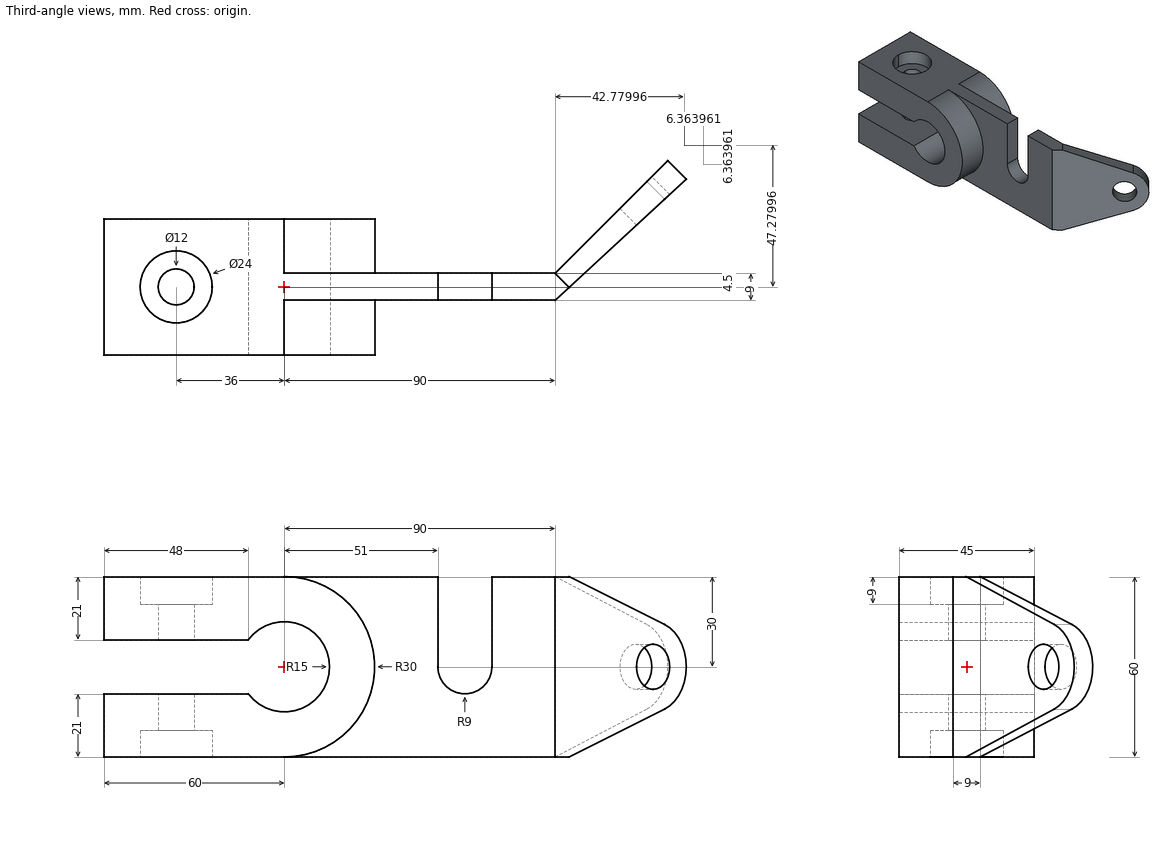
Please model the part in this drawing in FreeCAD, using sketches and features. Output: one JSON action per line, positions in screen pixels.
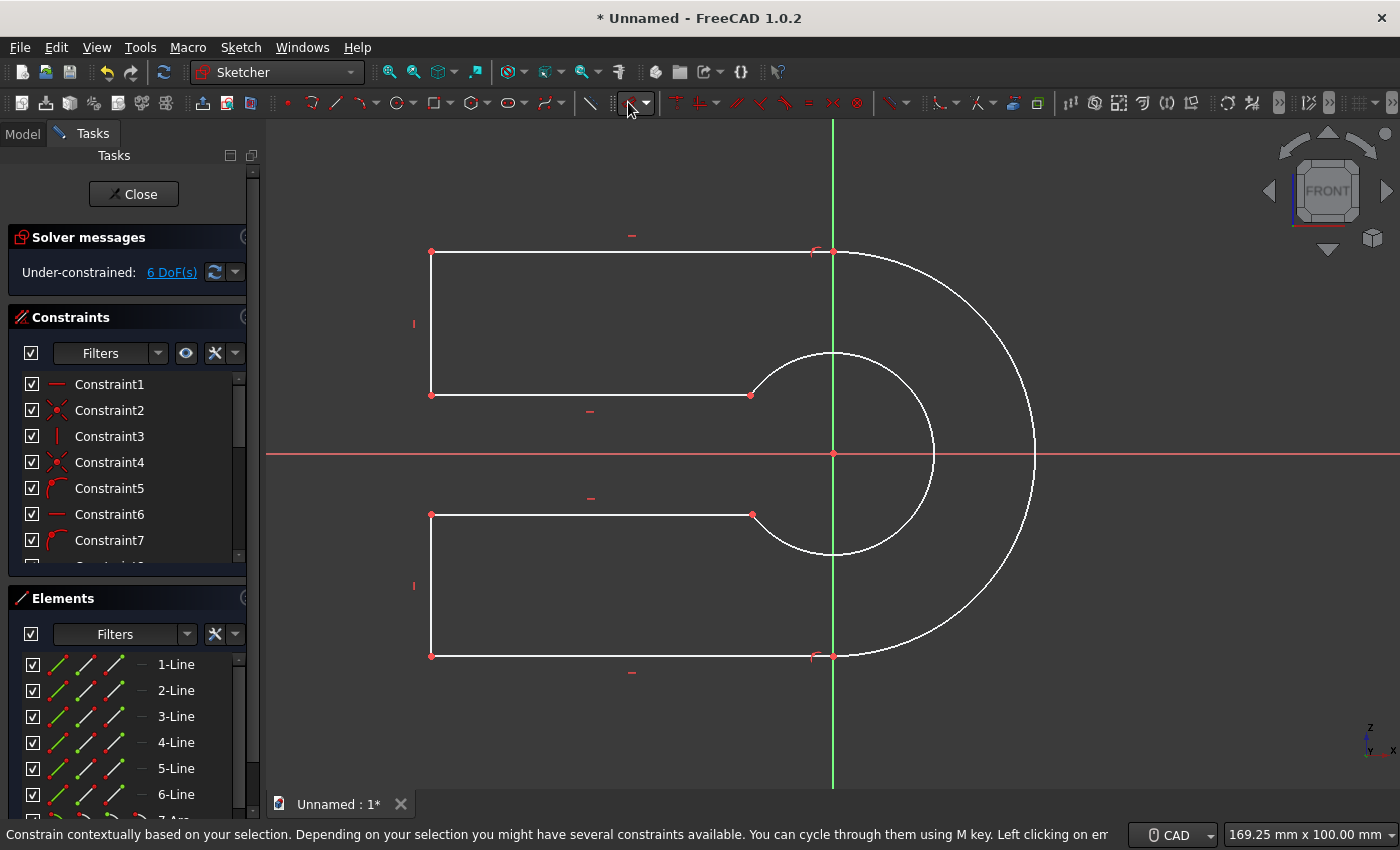
{"action": "left_click", "coordinate": [997, 573]}
{"action": "left_click", "coordinate": [1023, 592]}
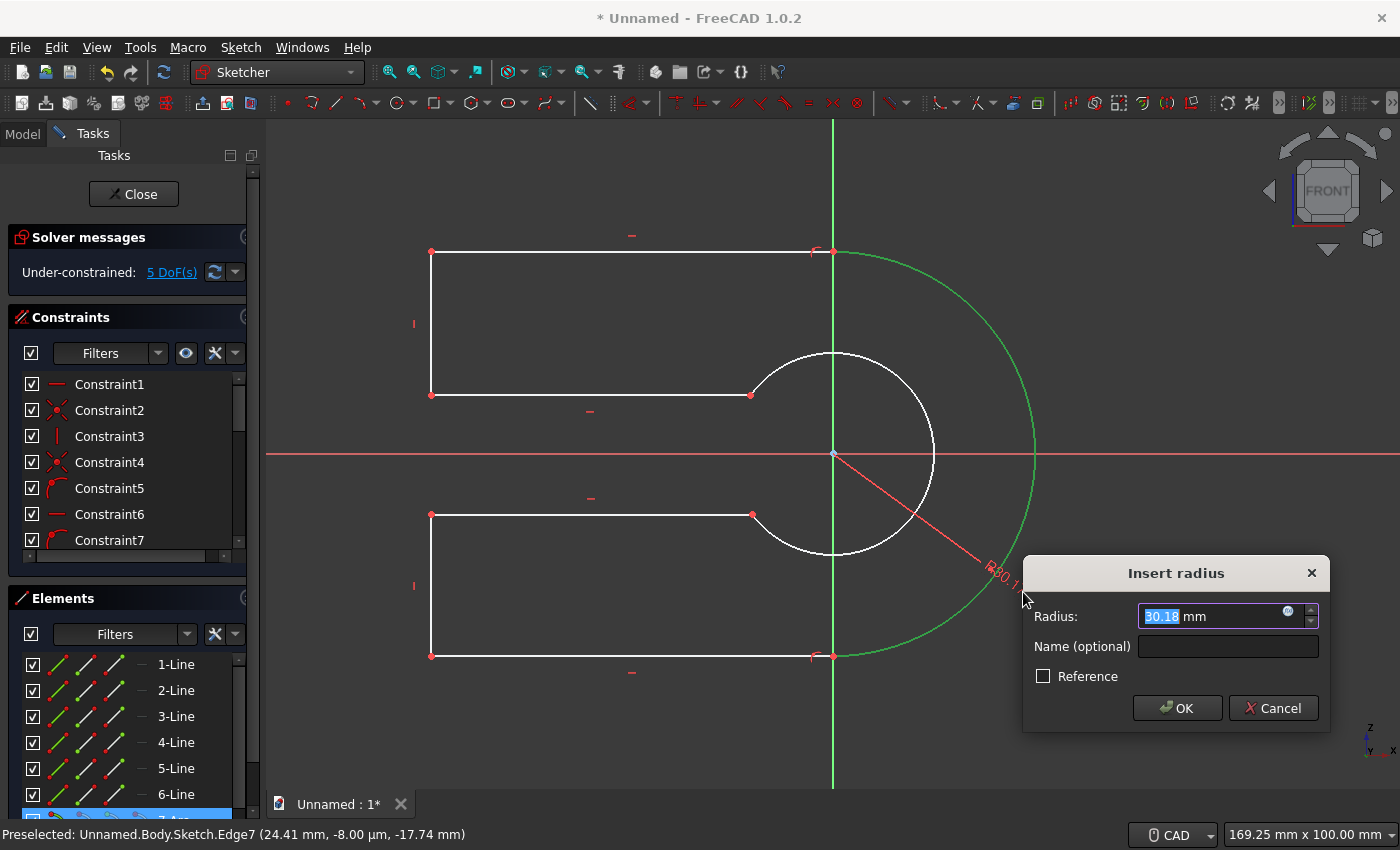
{"action": "type", "text": "30"}
{"action": "key", "text": "Return"}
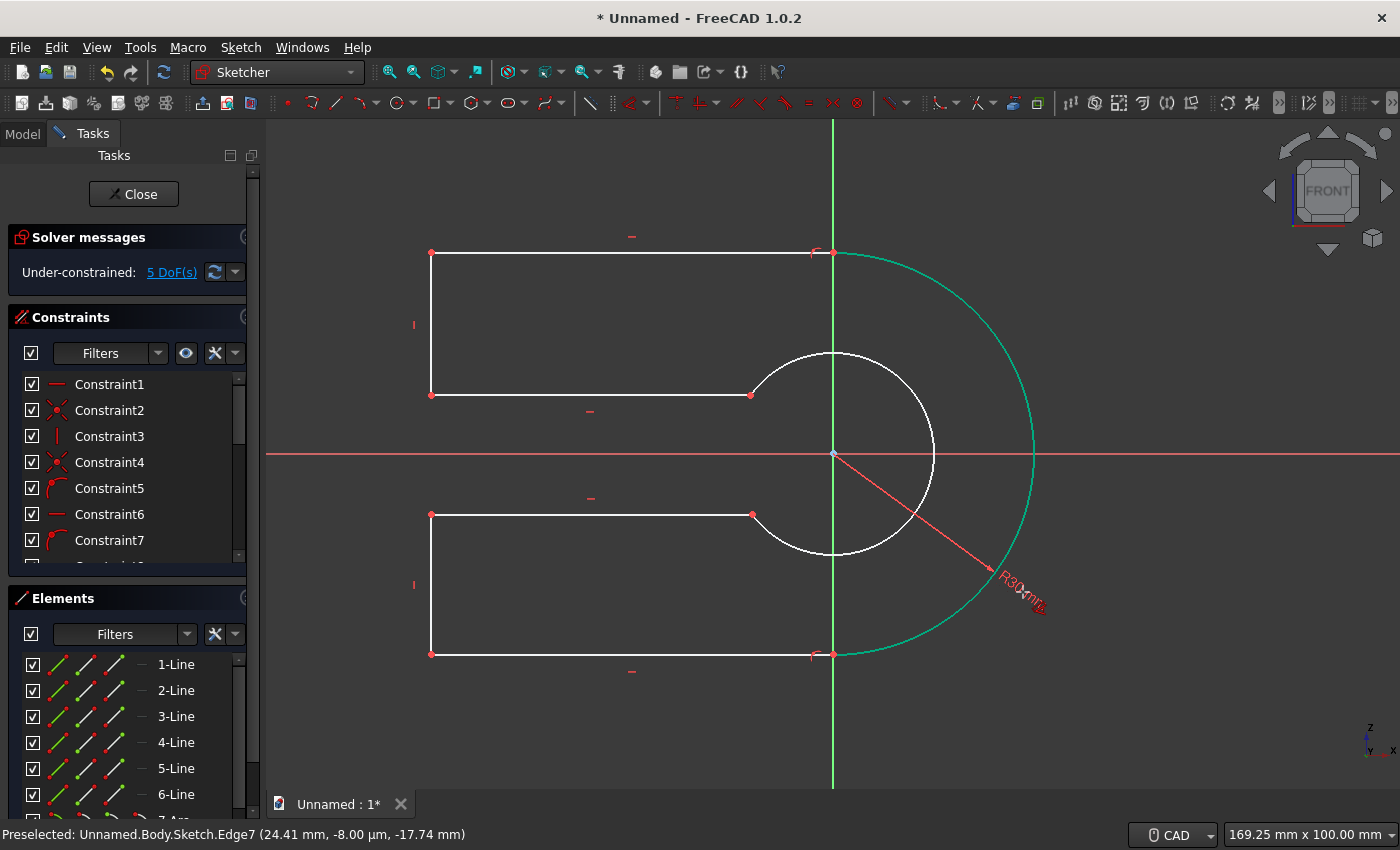
{"action": "left_click", "coordinate": [888, 539]}
{"action": "left_click", "coordinate": [905, 566]}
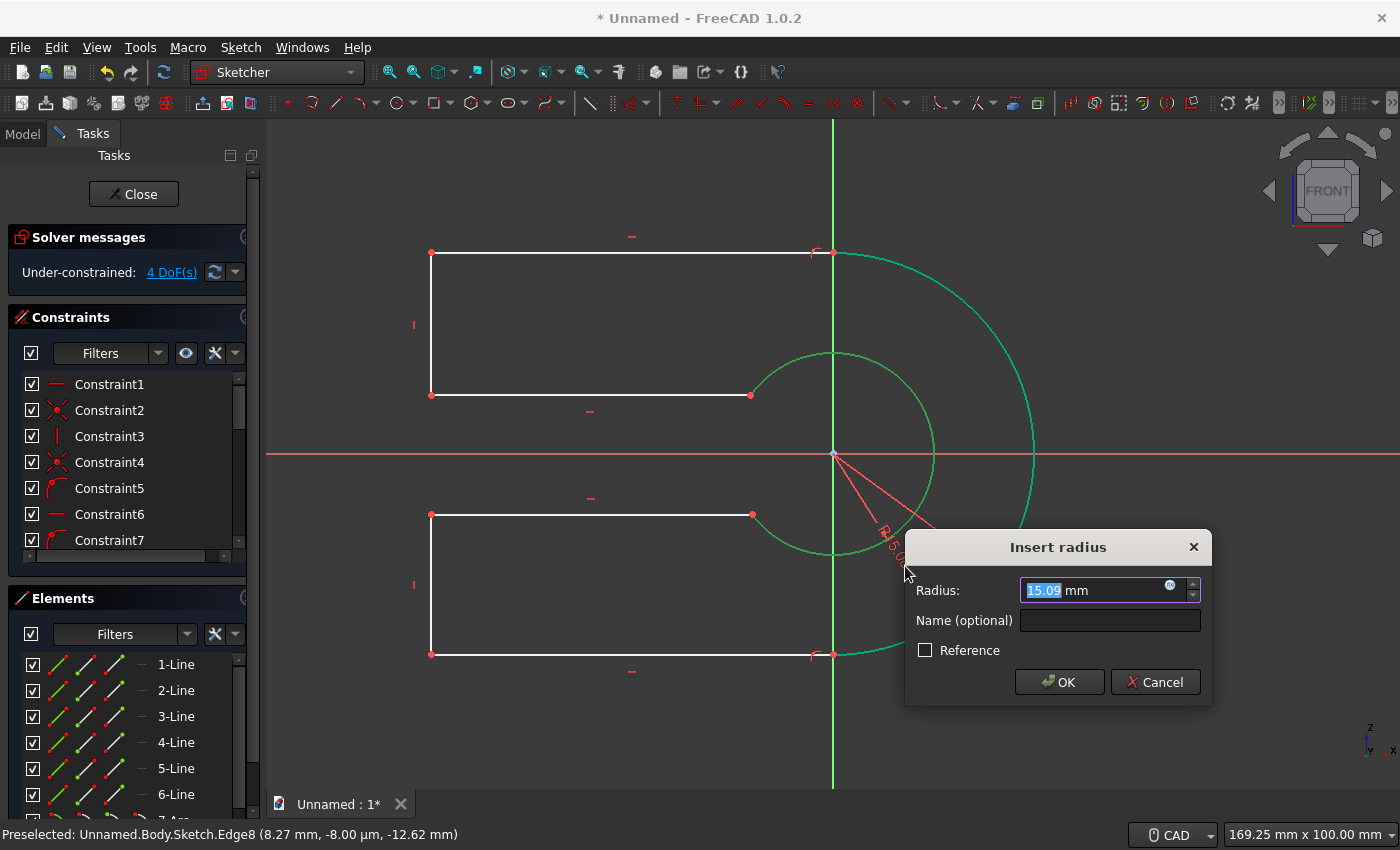
{"action": "type", "text": "15"}
{"action": "key", "text": "Return"}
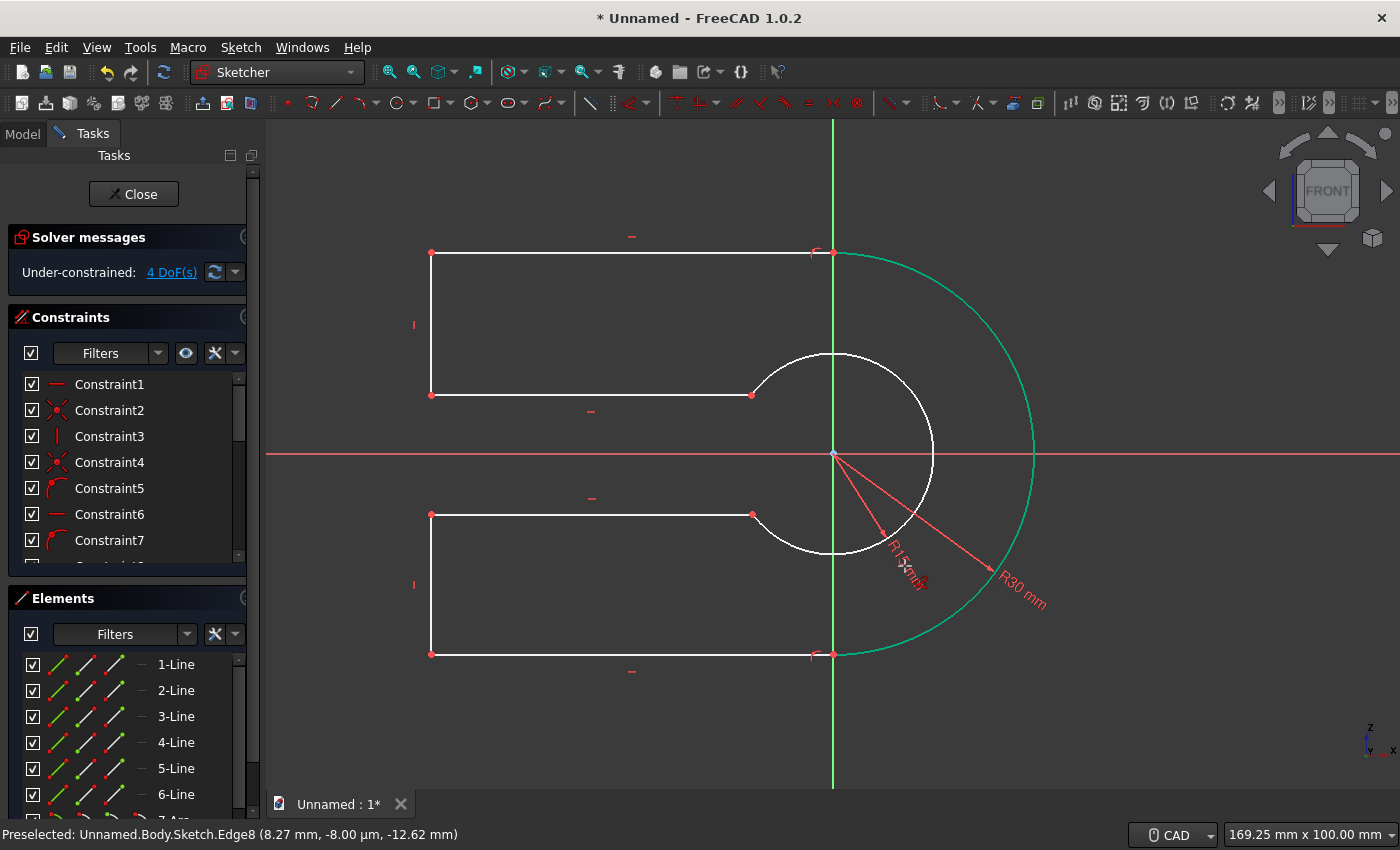
{"action": "left_click", "coordinate": [655, 395]}
{"action": "left_click", "coordinate": [591, 361]}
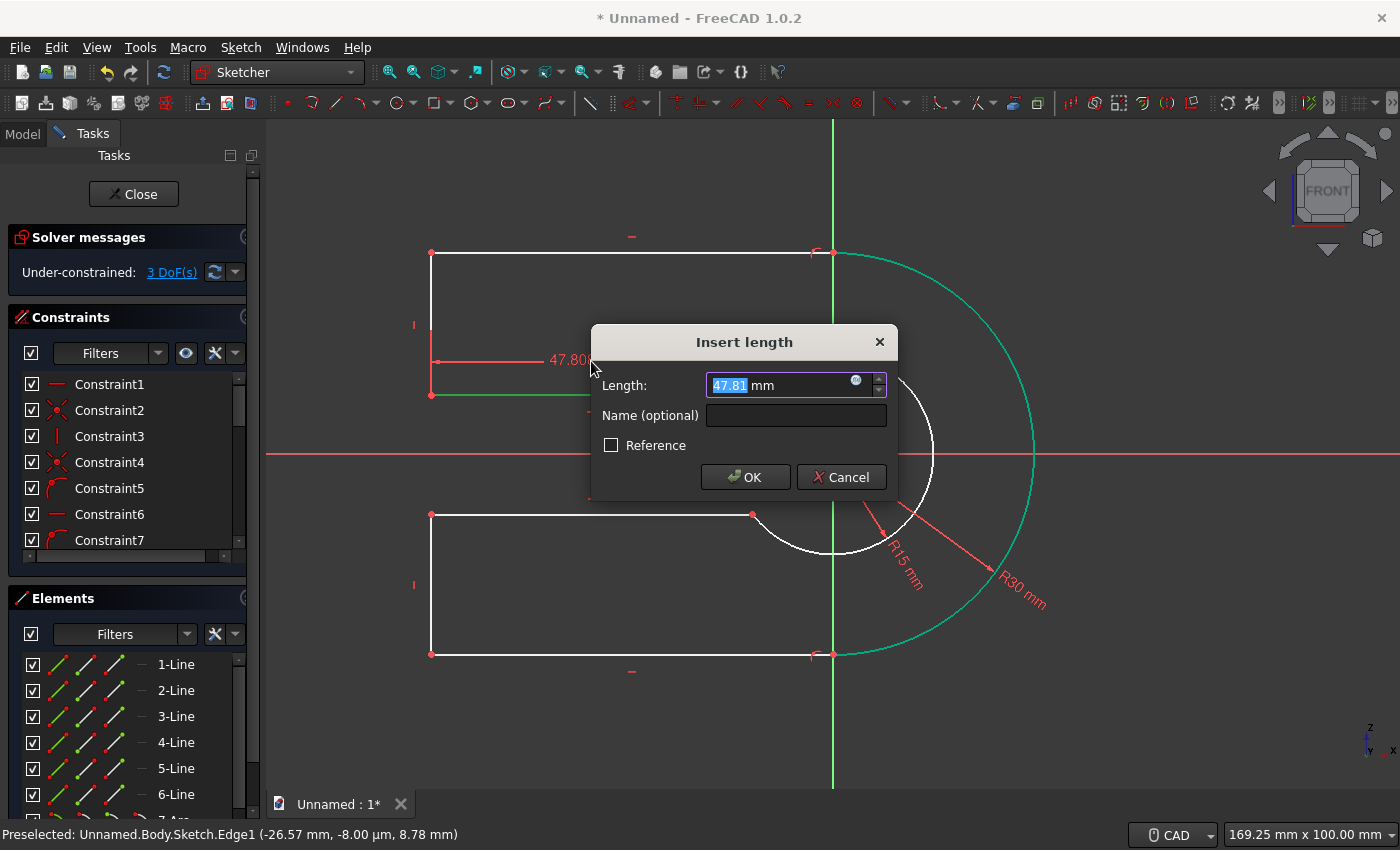
{"action": "type", "text": "48"}
{"action": "key", "text": "Return"}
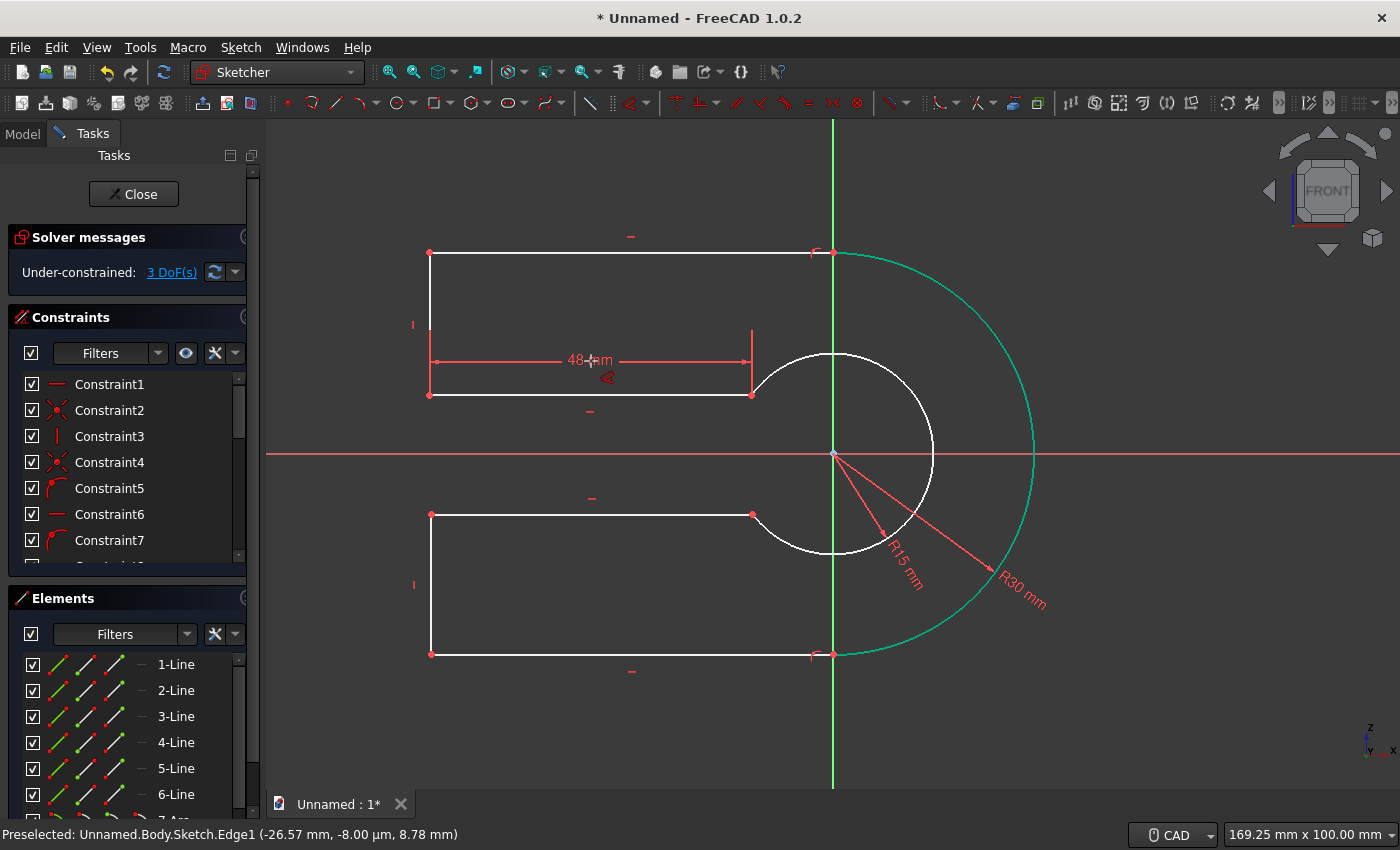
{"action": "left_click", "coordinate": [430, 353]}
{"action": "left_click", "coordinate": [396, 324]}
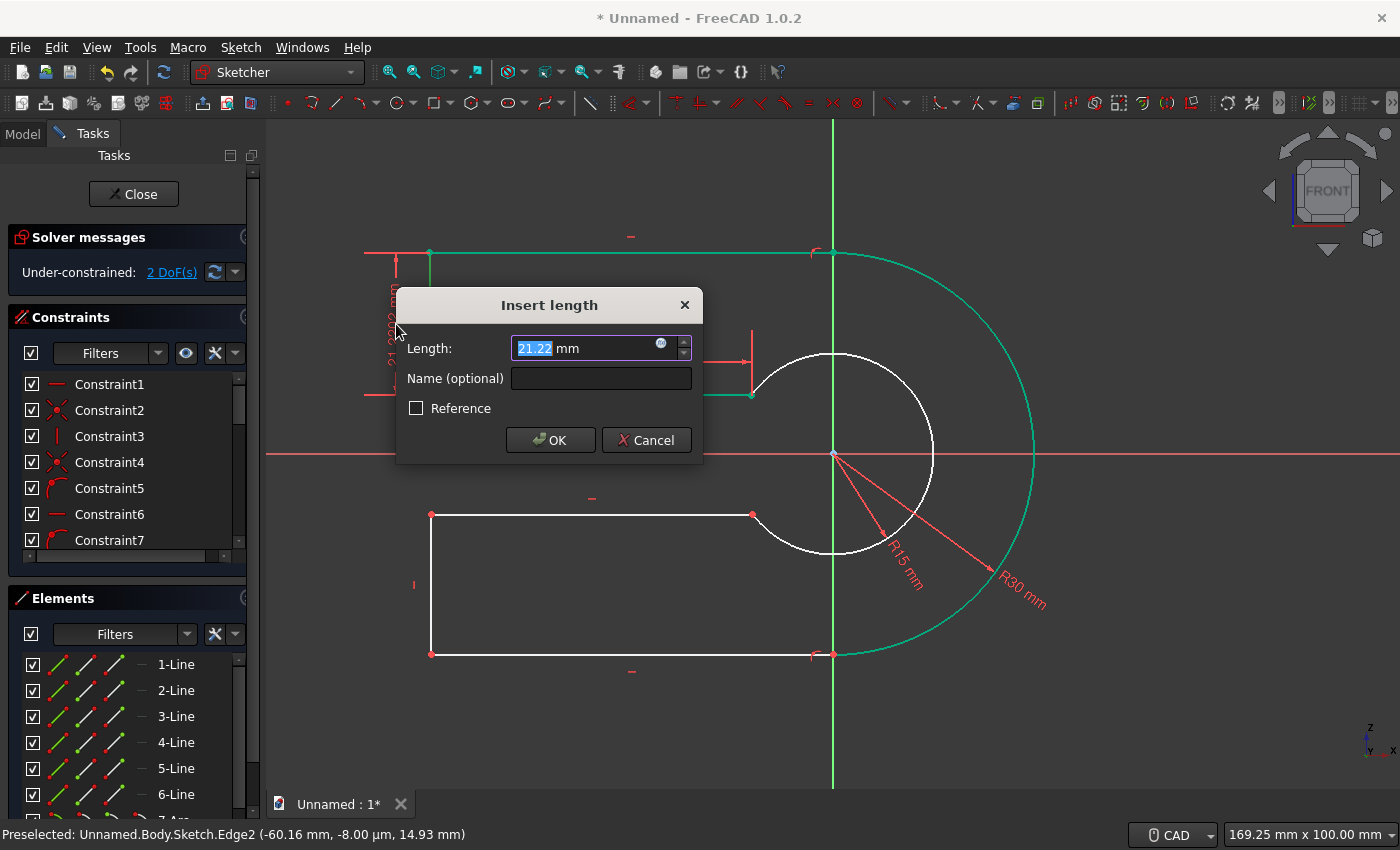
{"action": "type", "text": "21"}
{"action": "key", "text": "Return"}